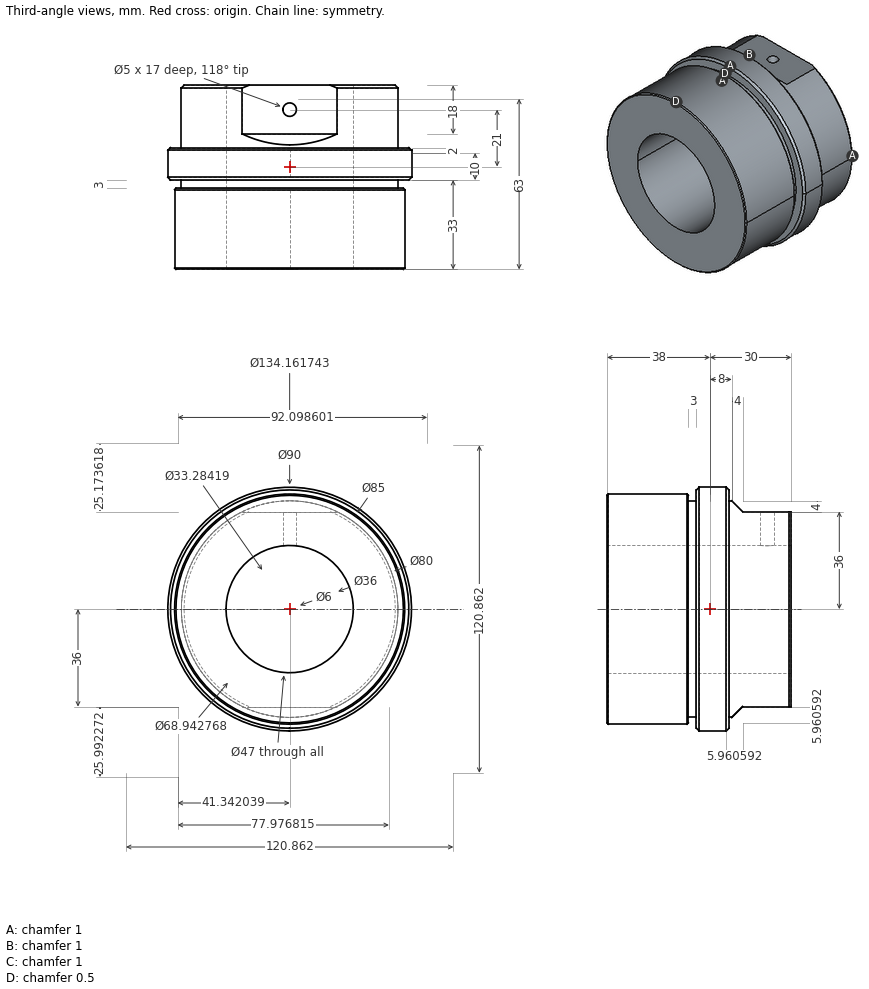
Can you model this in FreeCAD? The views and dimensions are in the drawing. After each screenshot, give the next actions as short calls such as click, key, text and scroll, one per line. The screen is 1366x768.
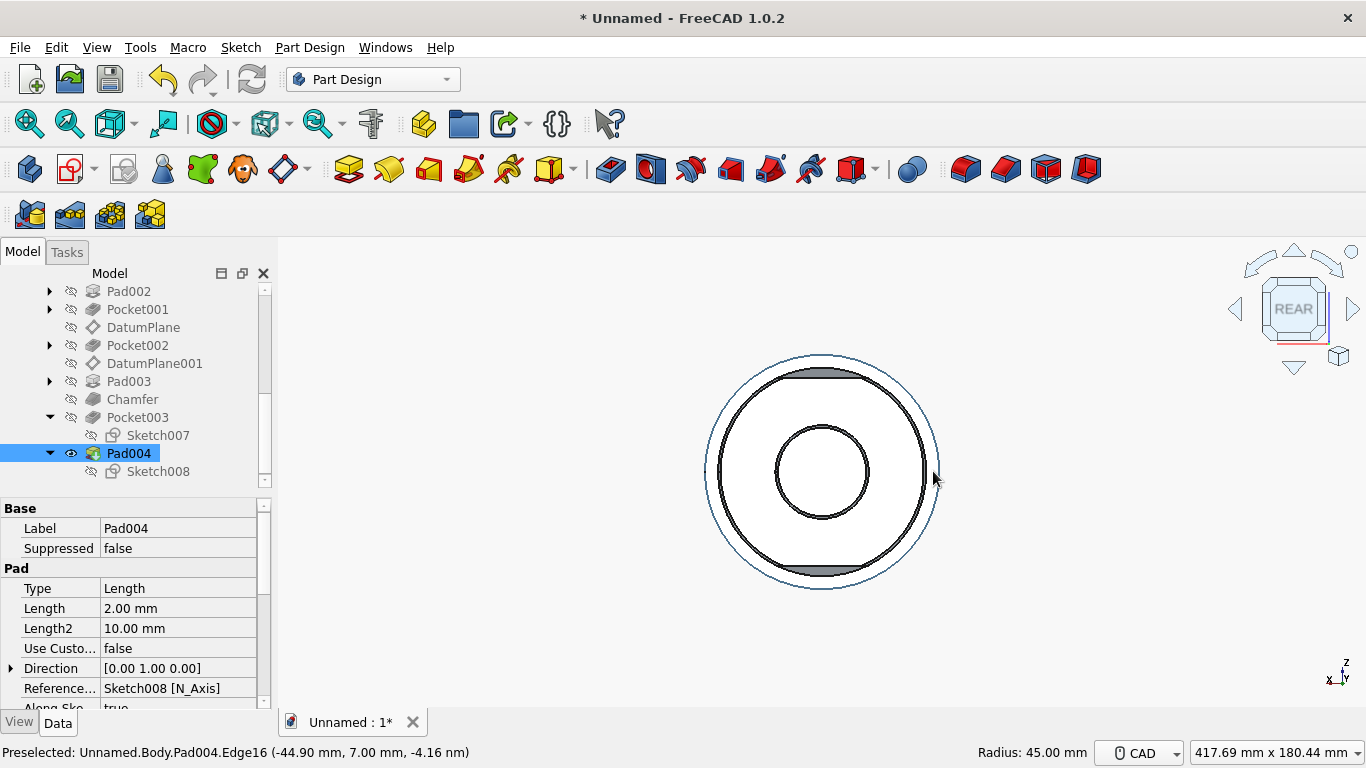
click(1006, 170)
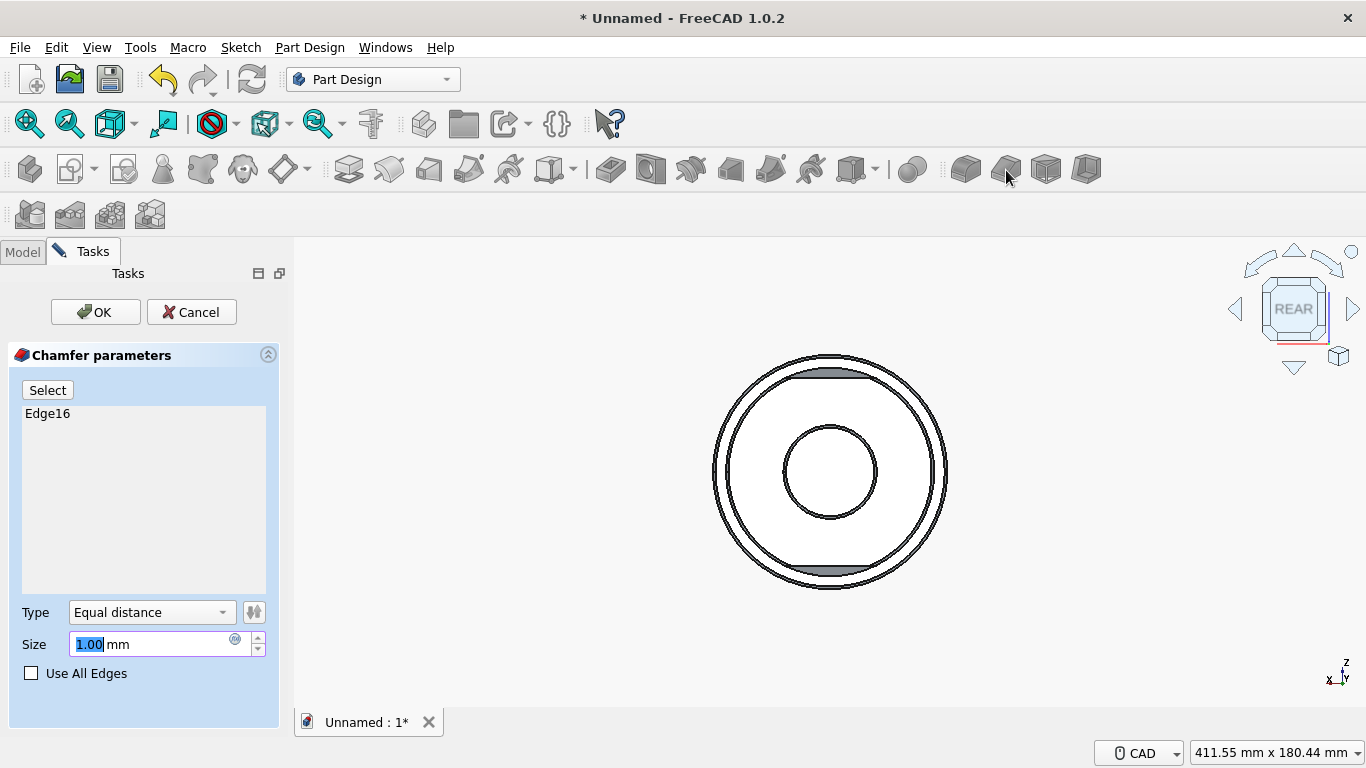
text(1)
key(Tab)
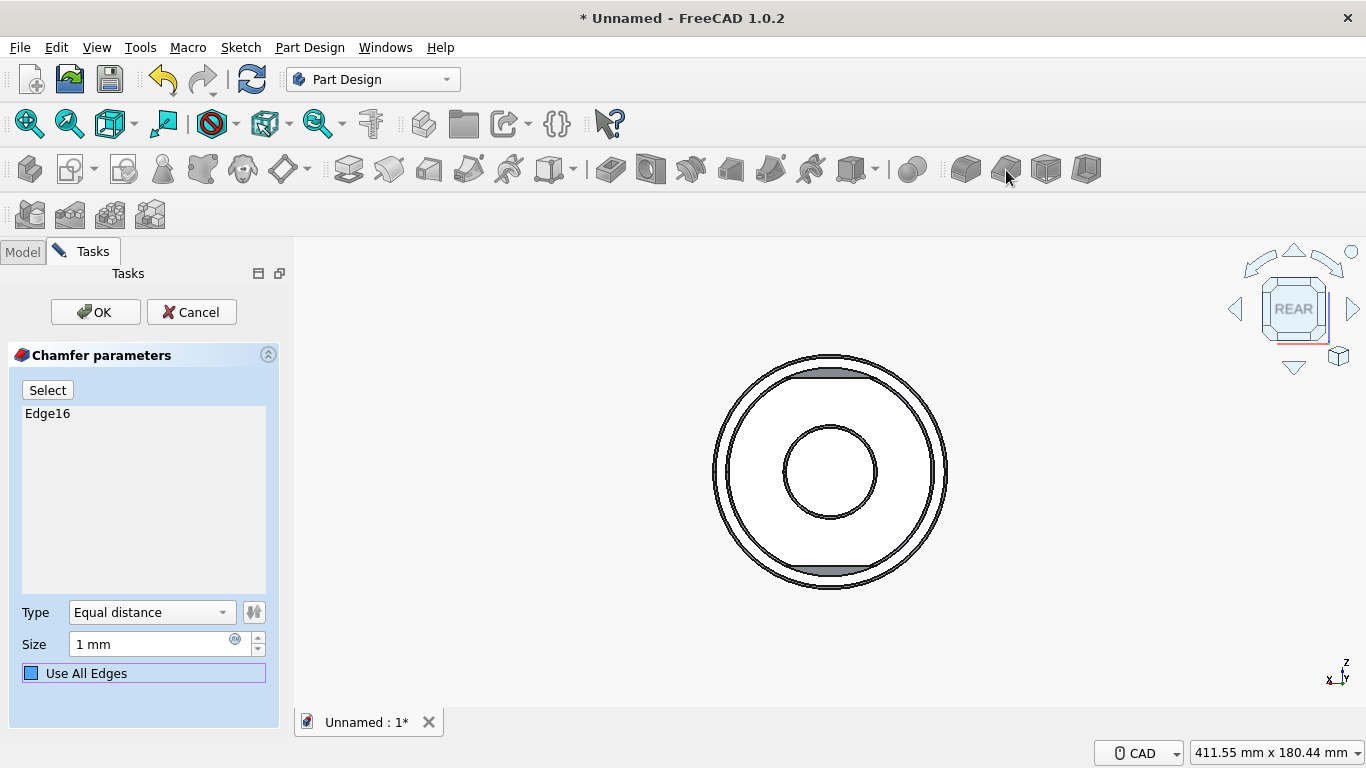
click(96, 312)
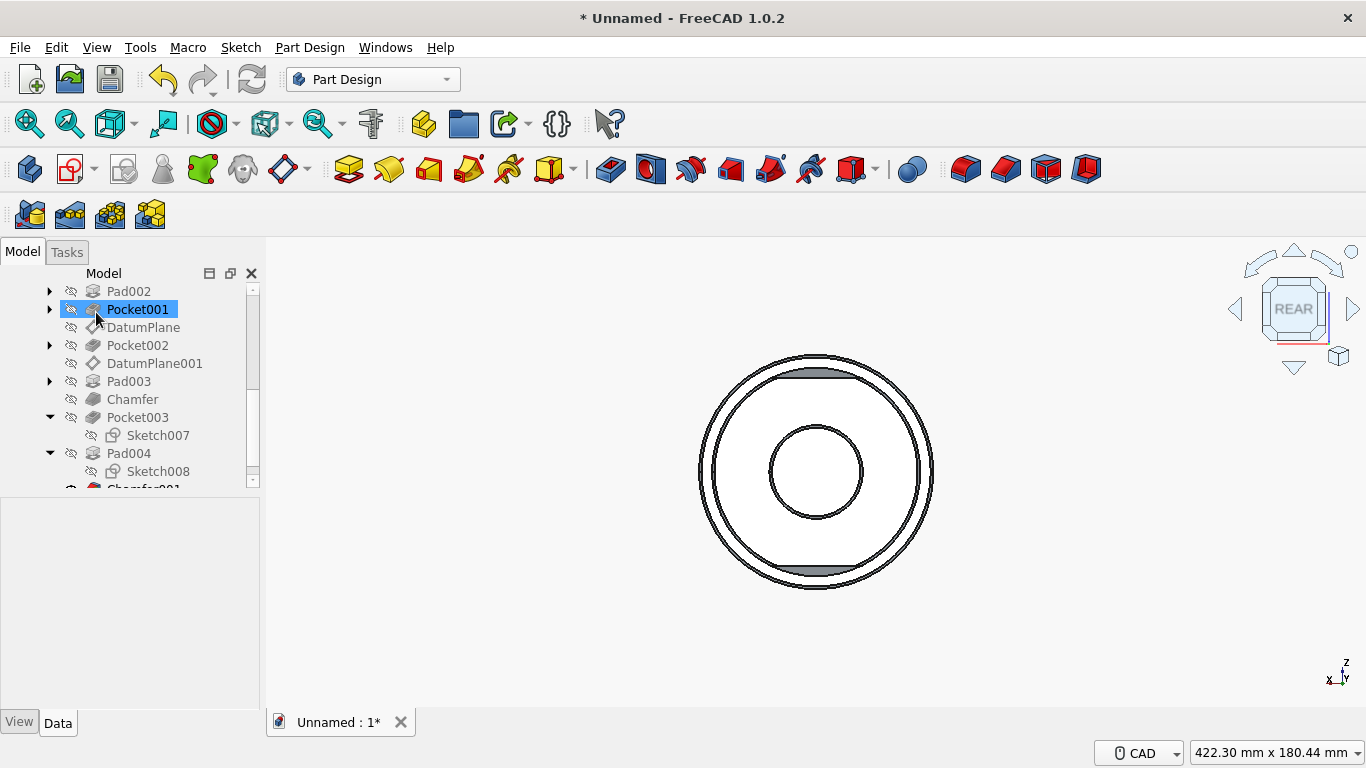
key(0)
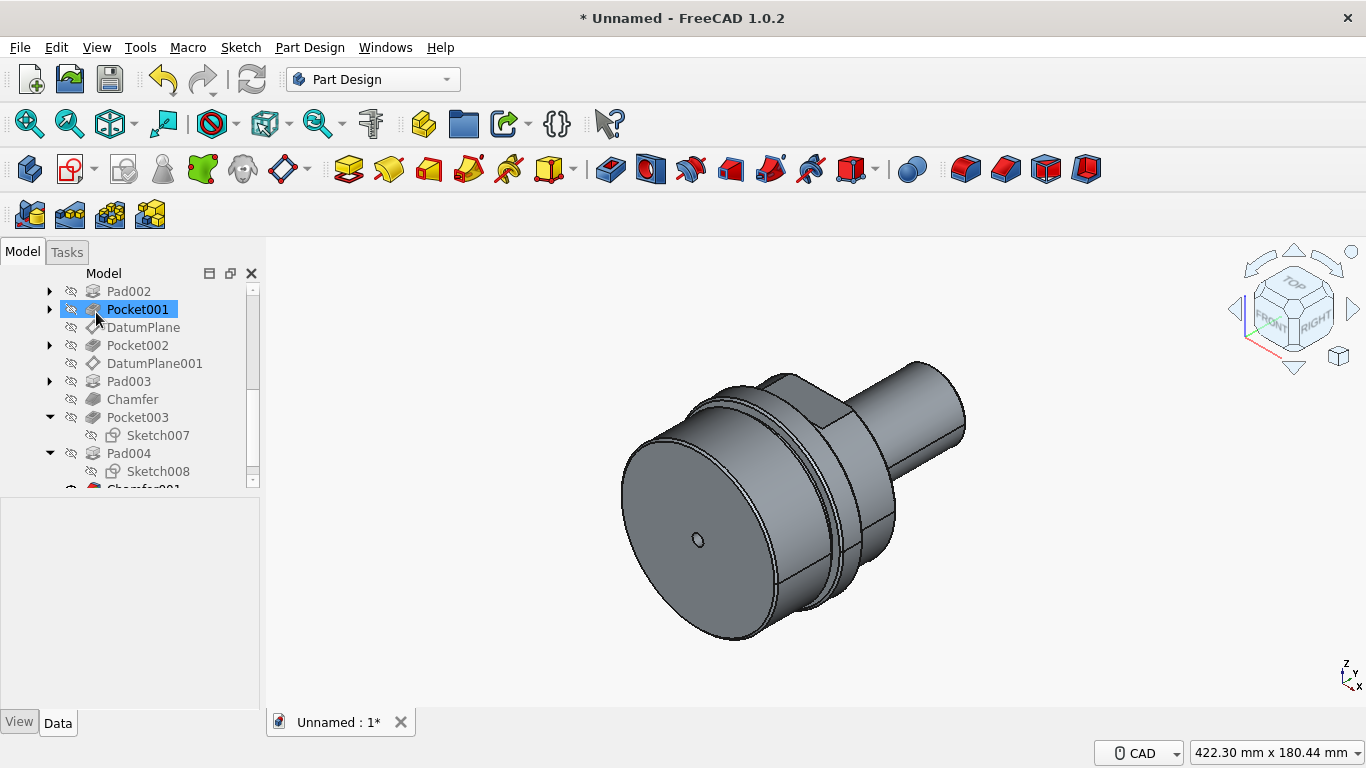
click(777, 435)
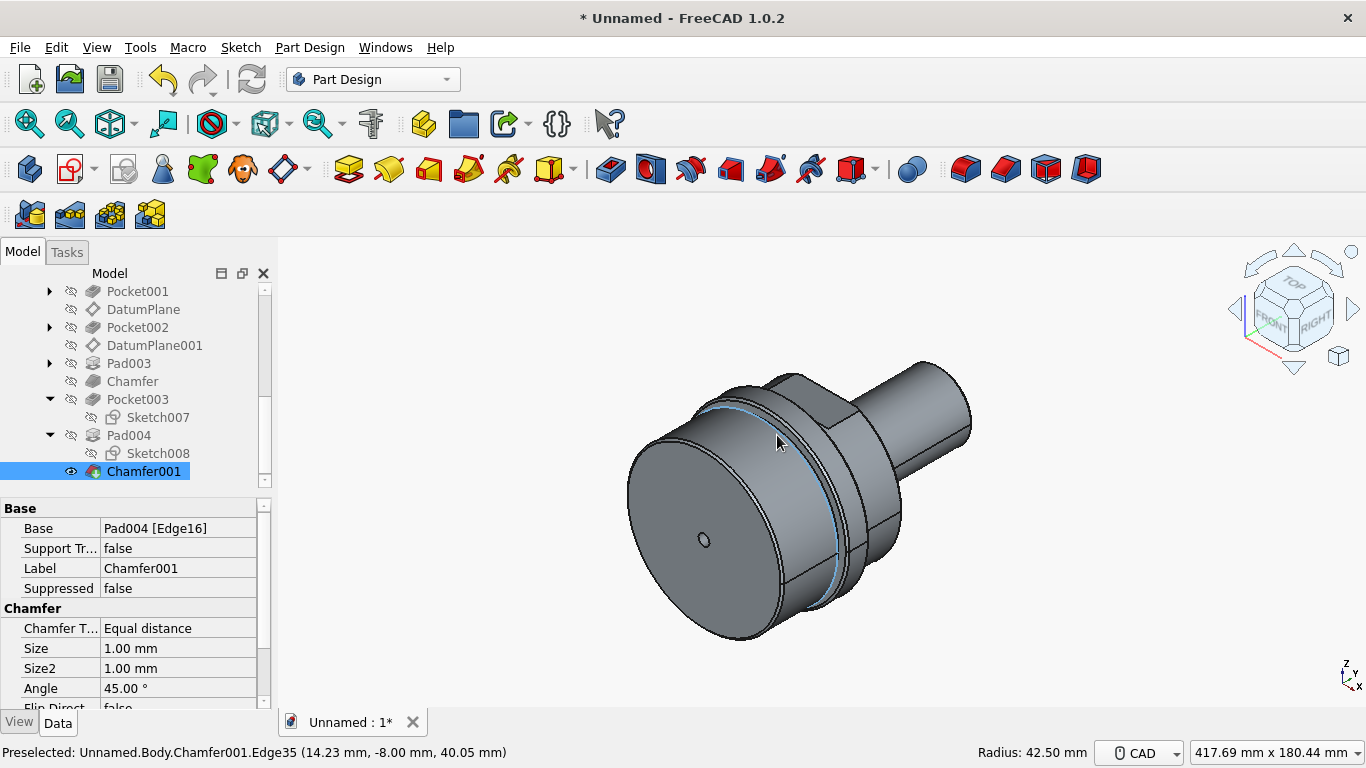
click(1006, 170)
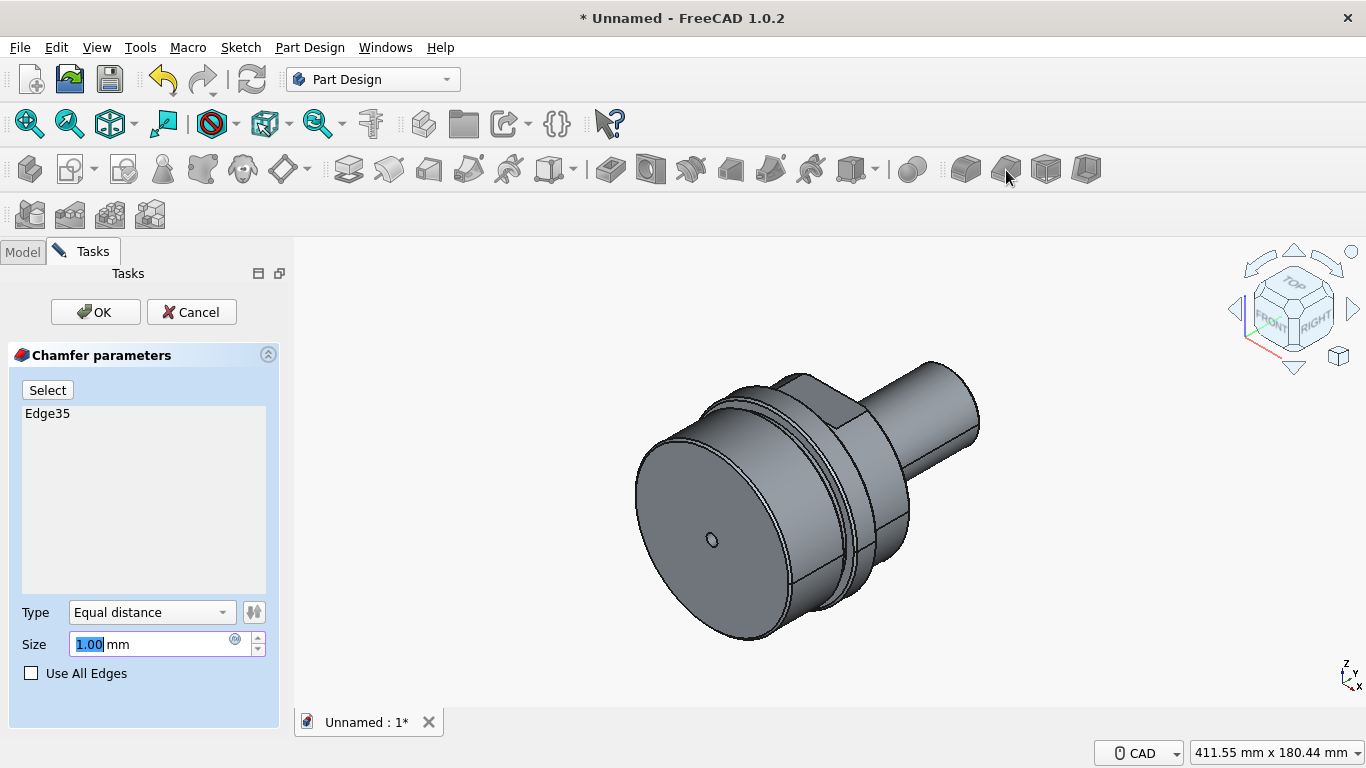
text(1)
key(Tab)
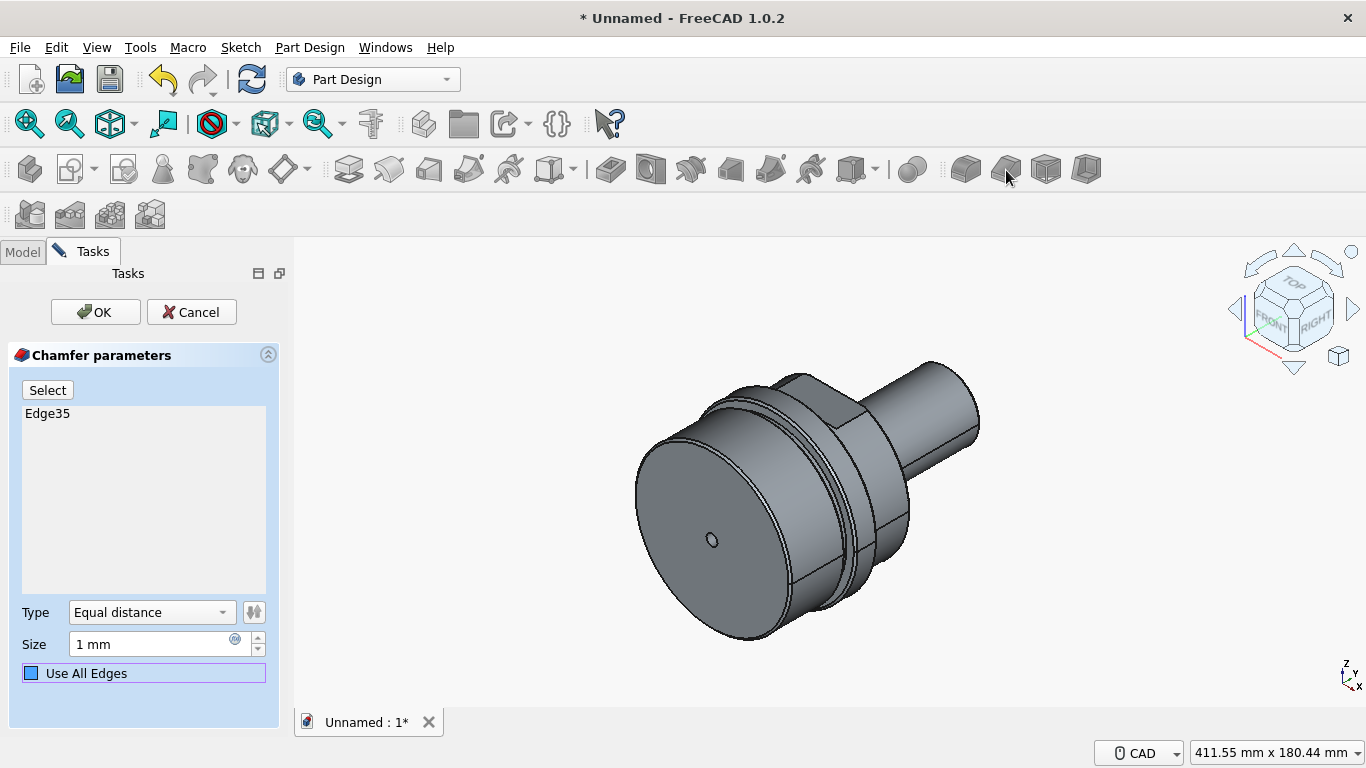
click(96, 312)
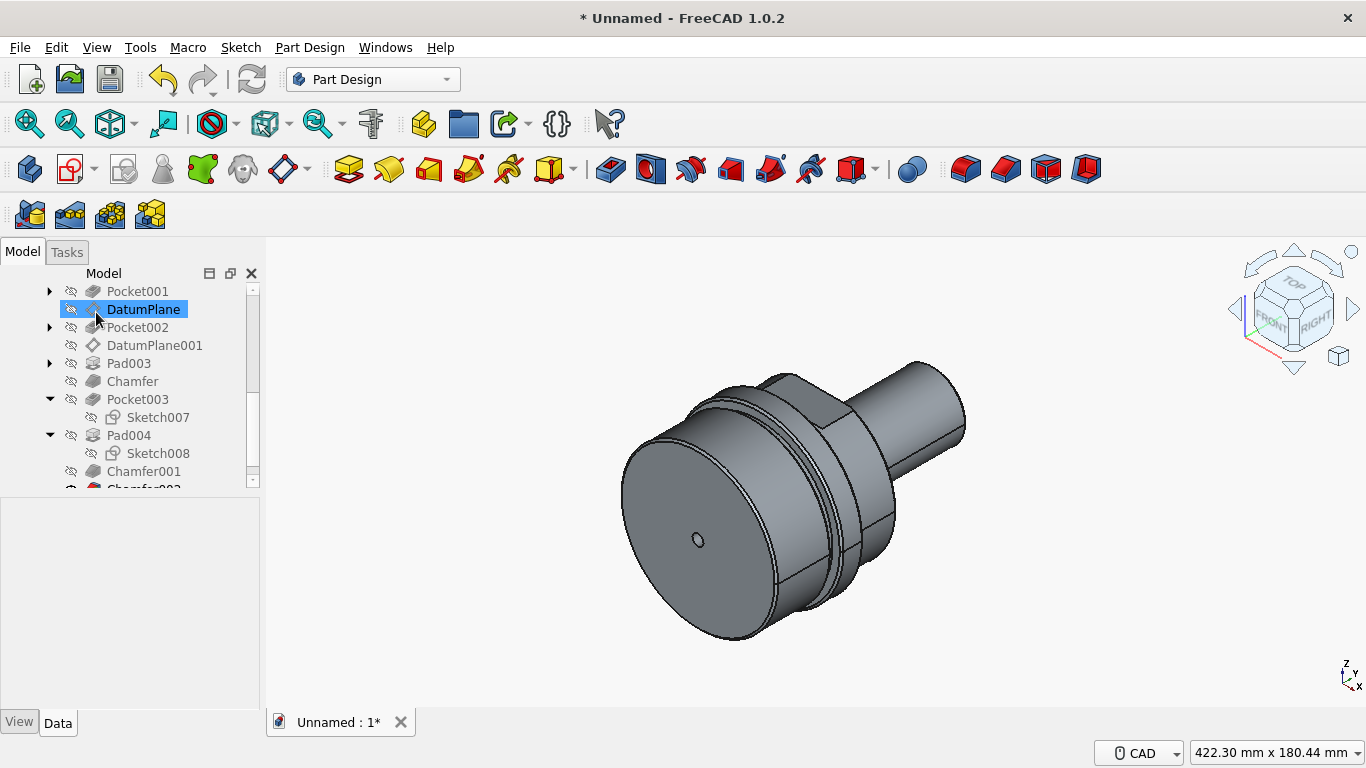
key(1)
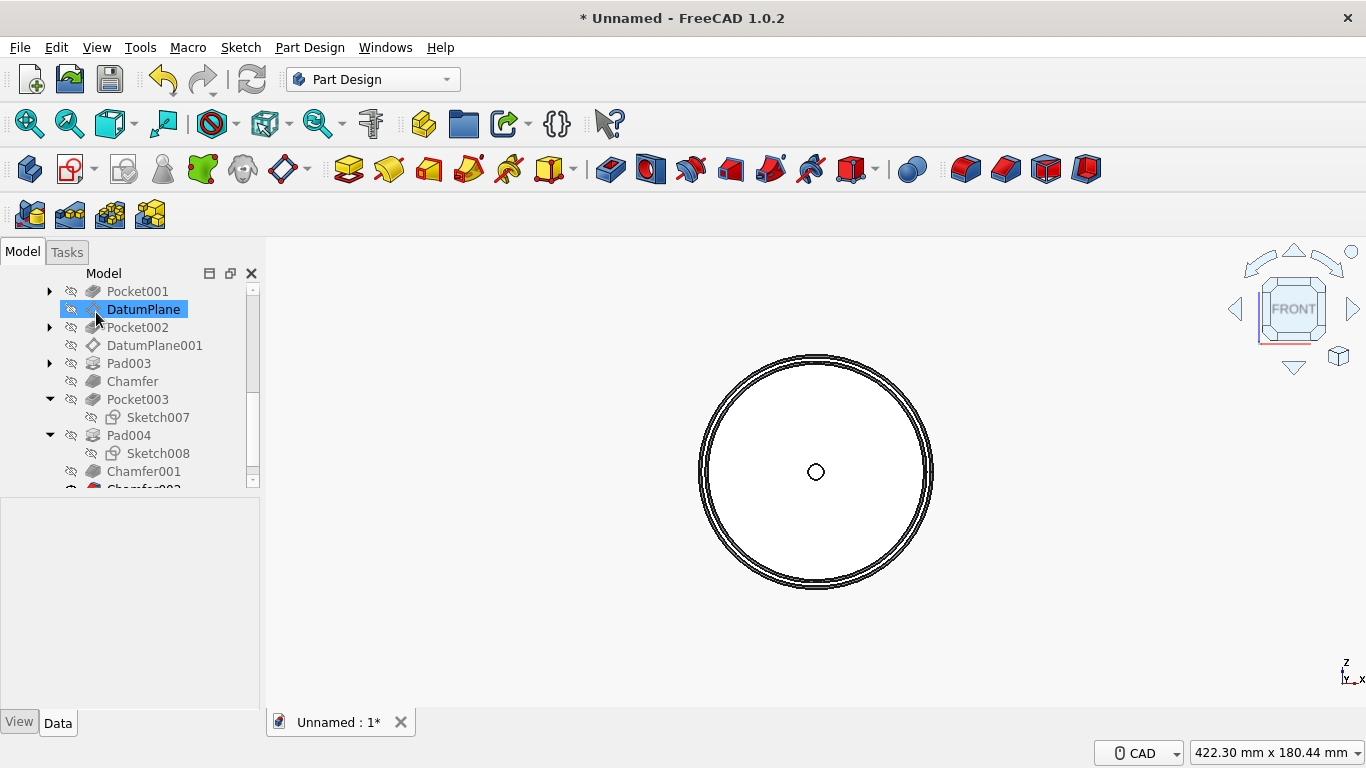
key(0)